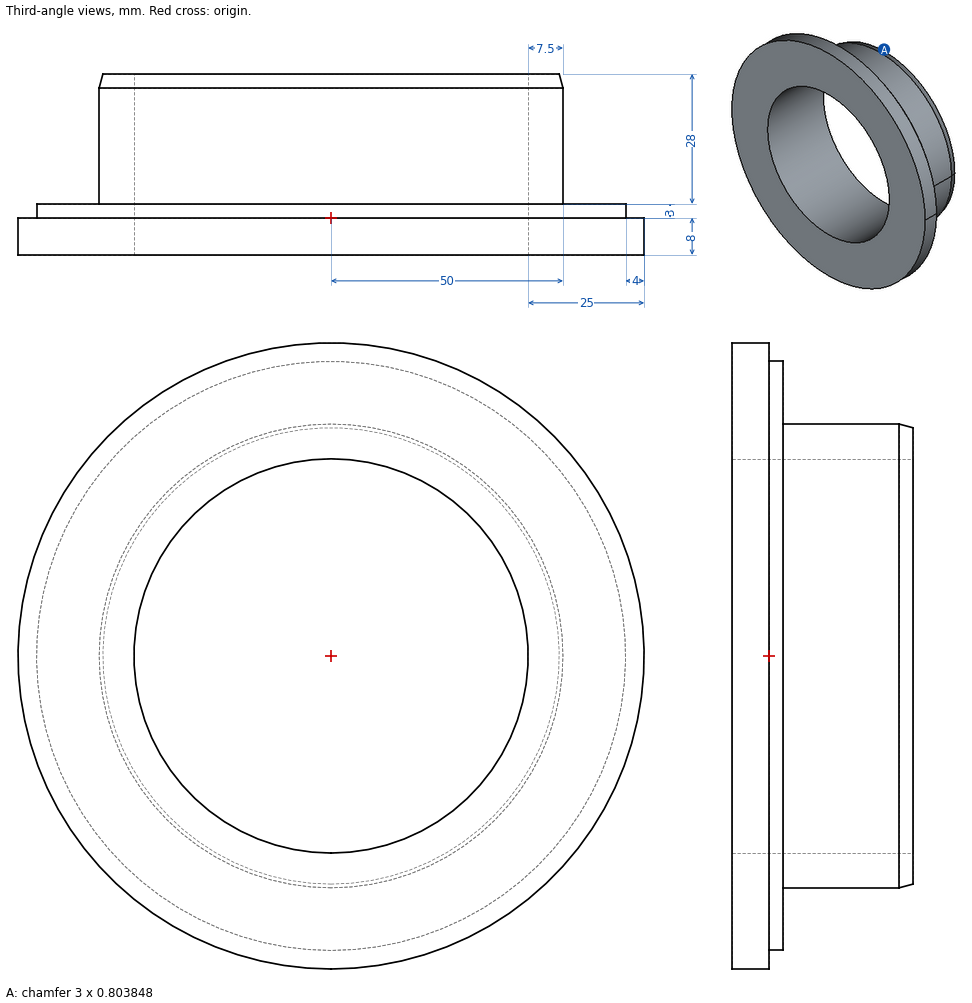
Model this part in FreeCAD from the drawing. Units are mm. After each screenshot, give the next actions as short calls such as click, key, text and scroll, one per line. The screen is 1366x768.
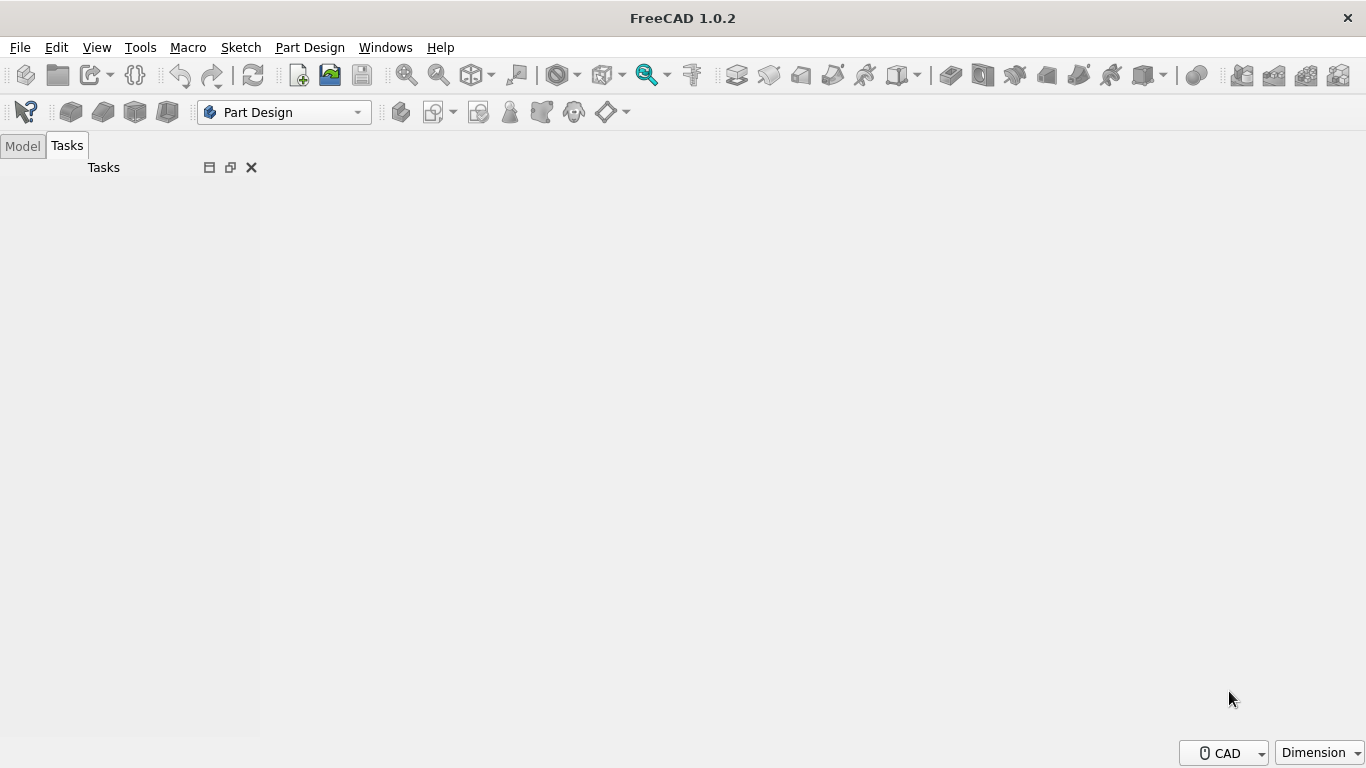
click(298, 76)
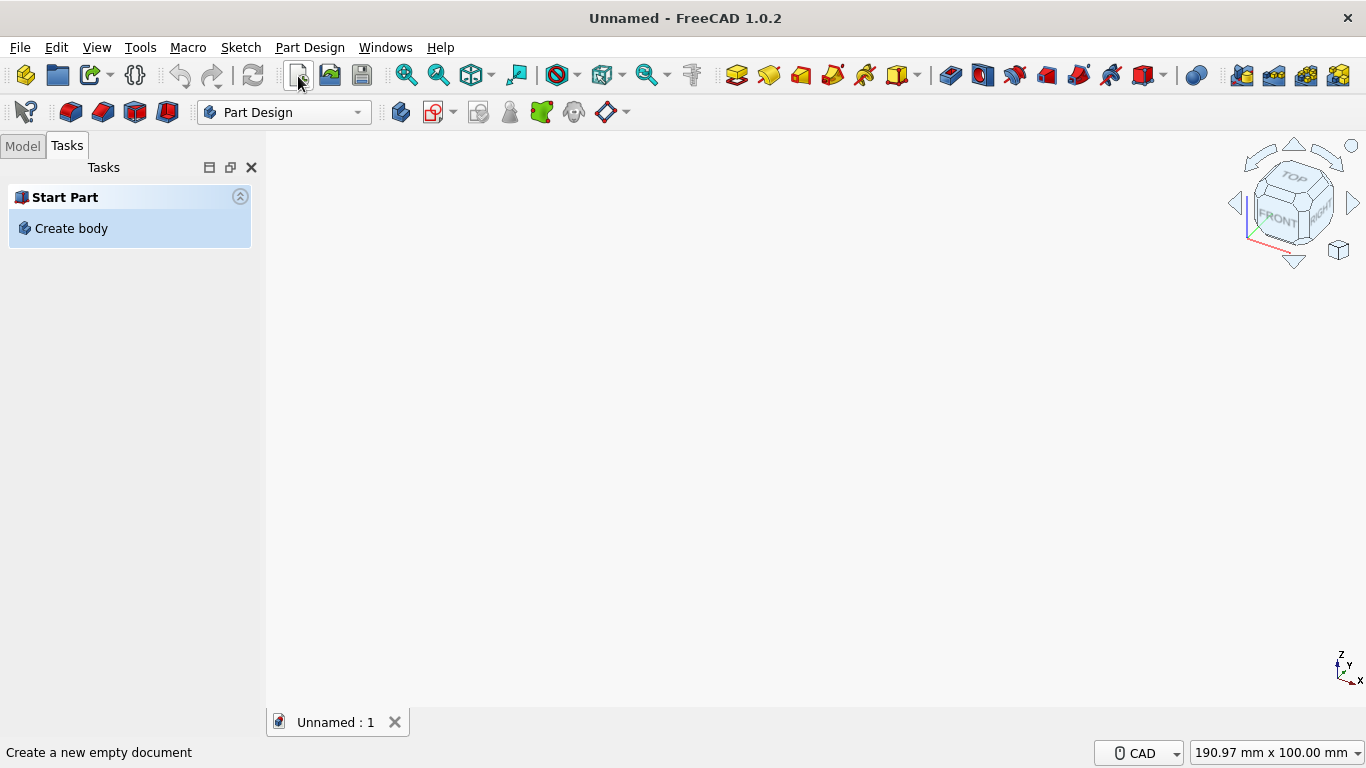
click(434, 112)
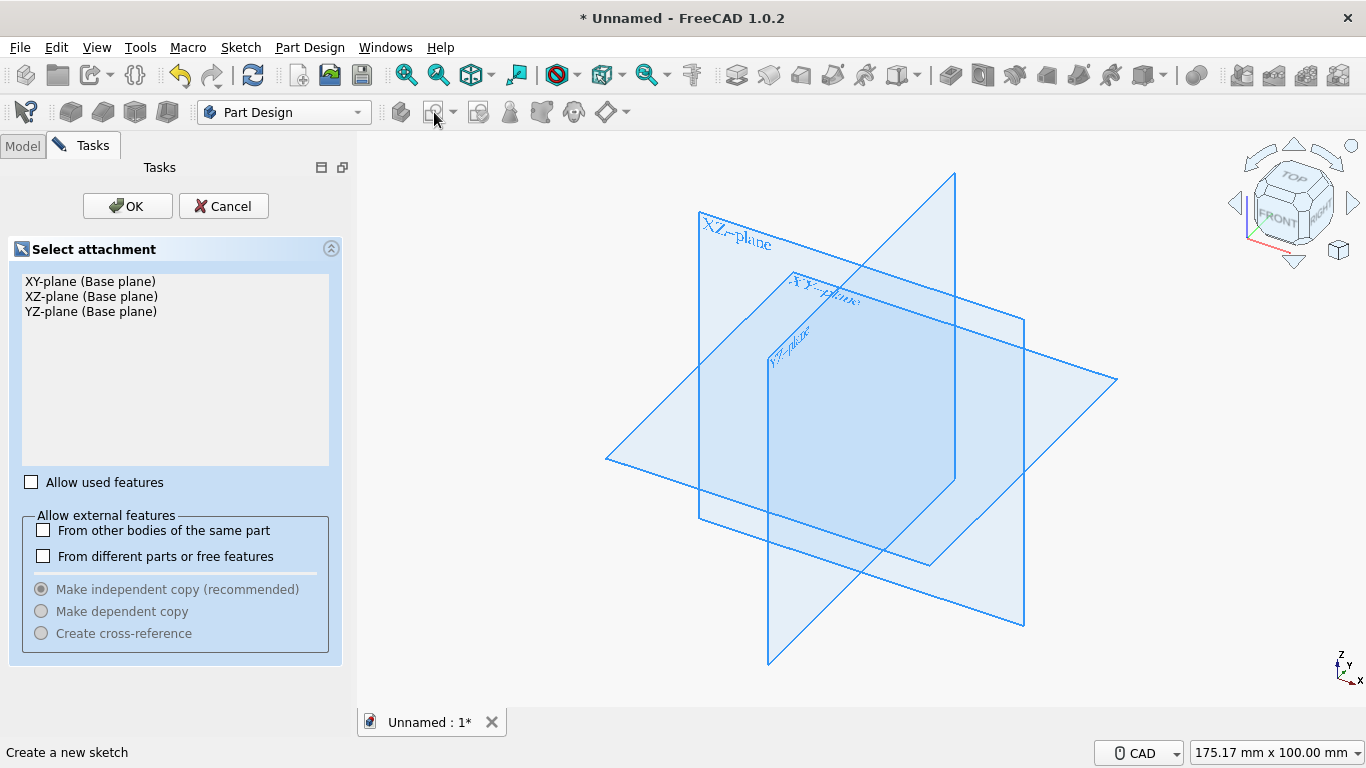
click(82, 282)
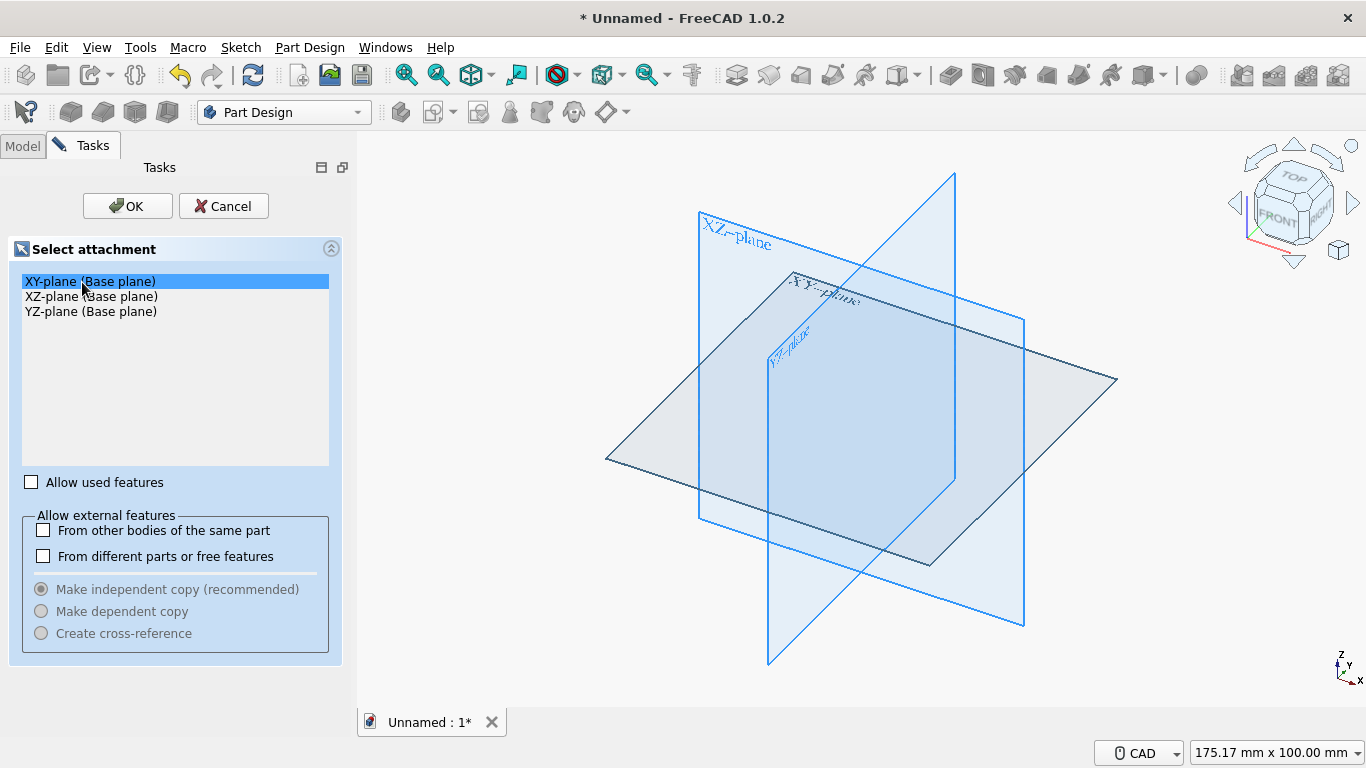
click(128, 206)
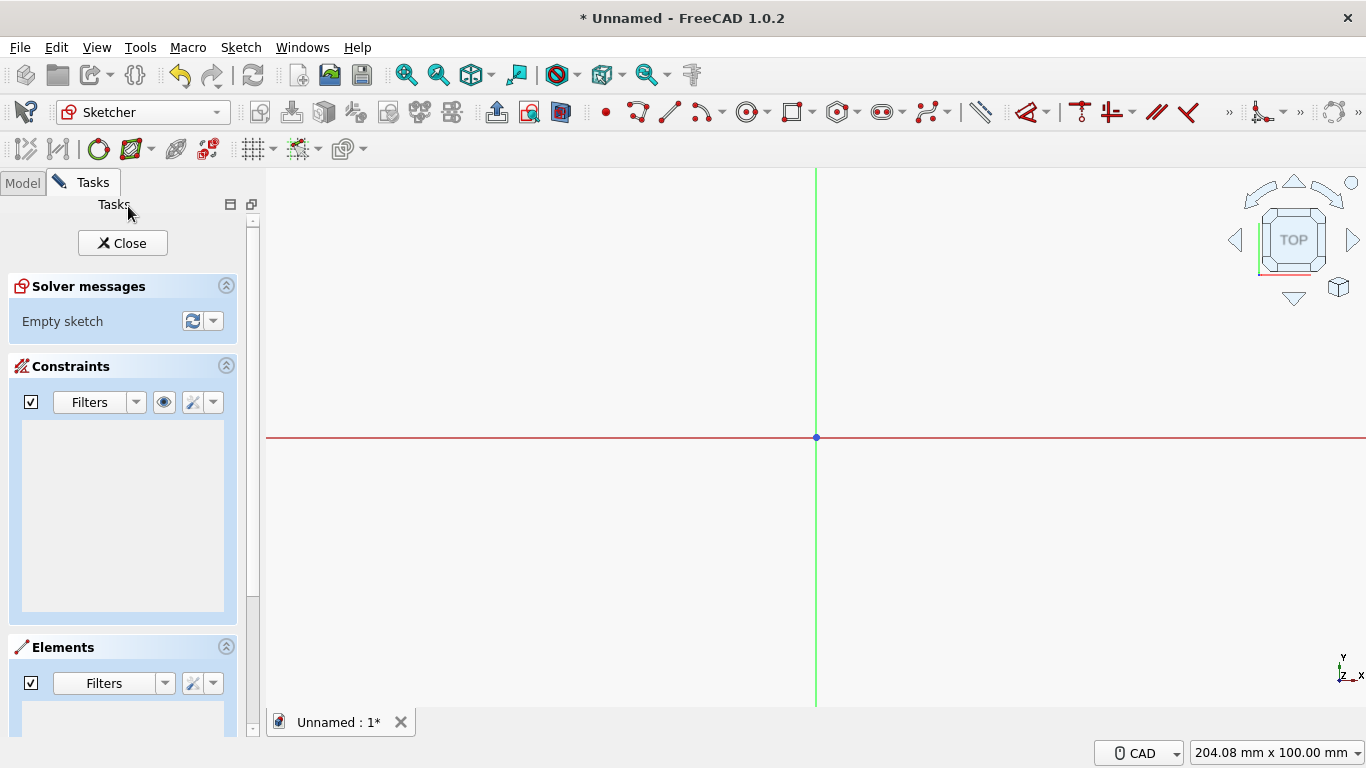
scroll(1201, 249, up, 2)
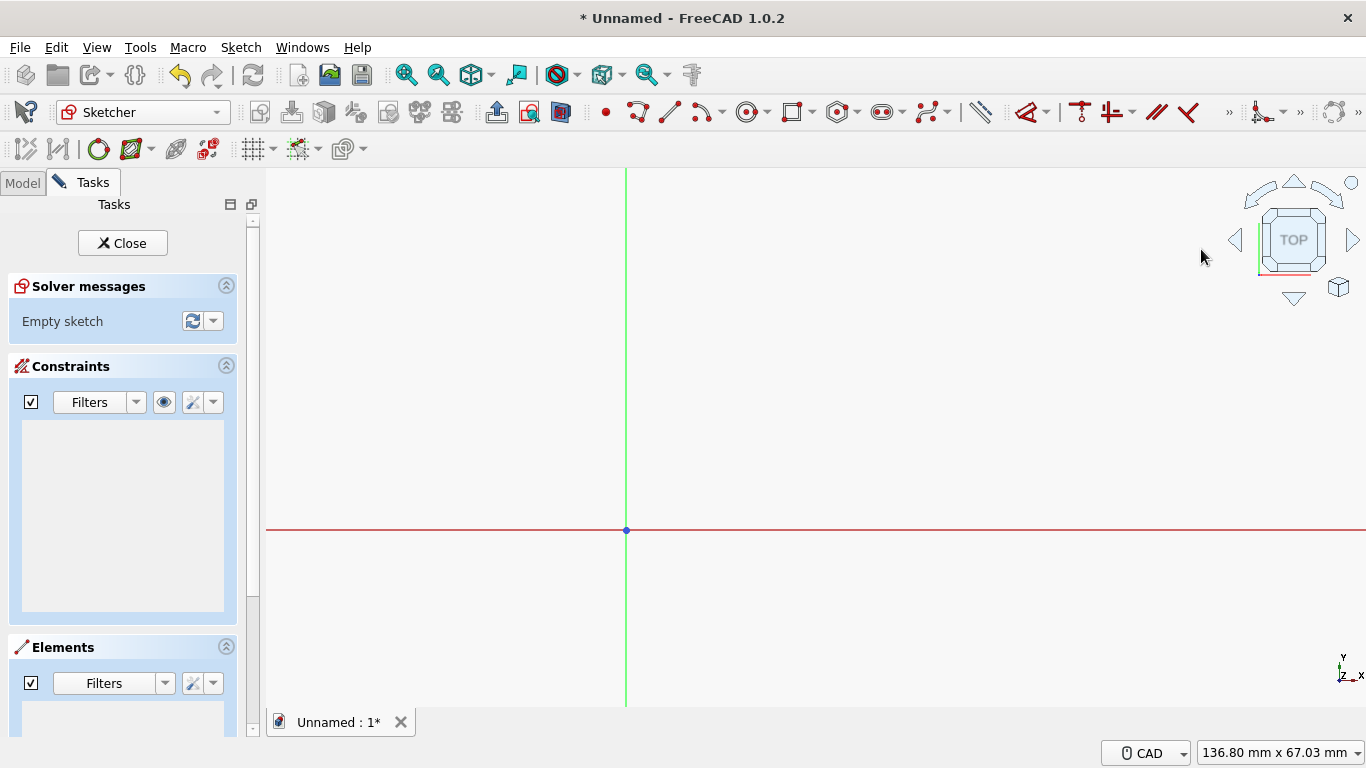
click(638, 112)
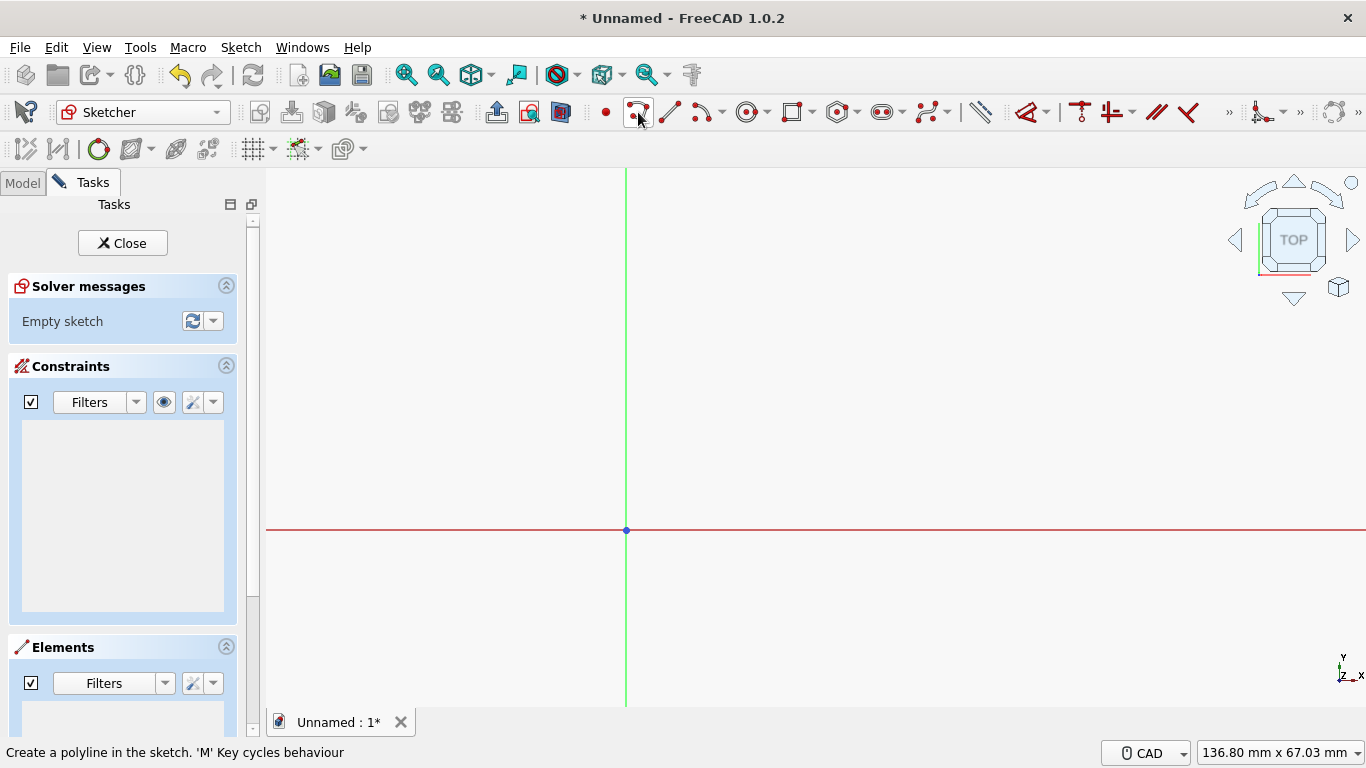
click(968, 594)
click(1169, 594)
click(1169, 530)
click(1137, 521)
click(1137, 506)
click(1028, 506)
click(1028, 281)
click(968, 281)
click(968, 595)
key(Escape)
key(Escape)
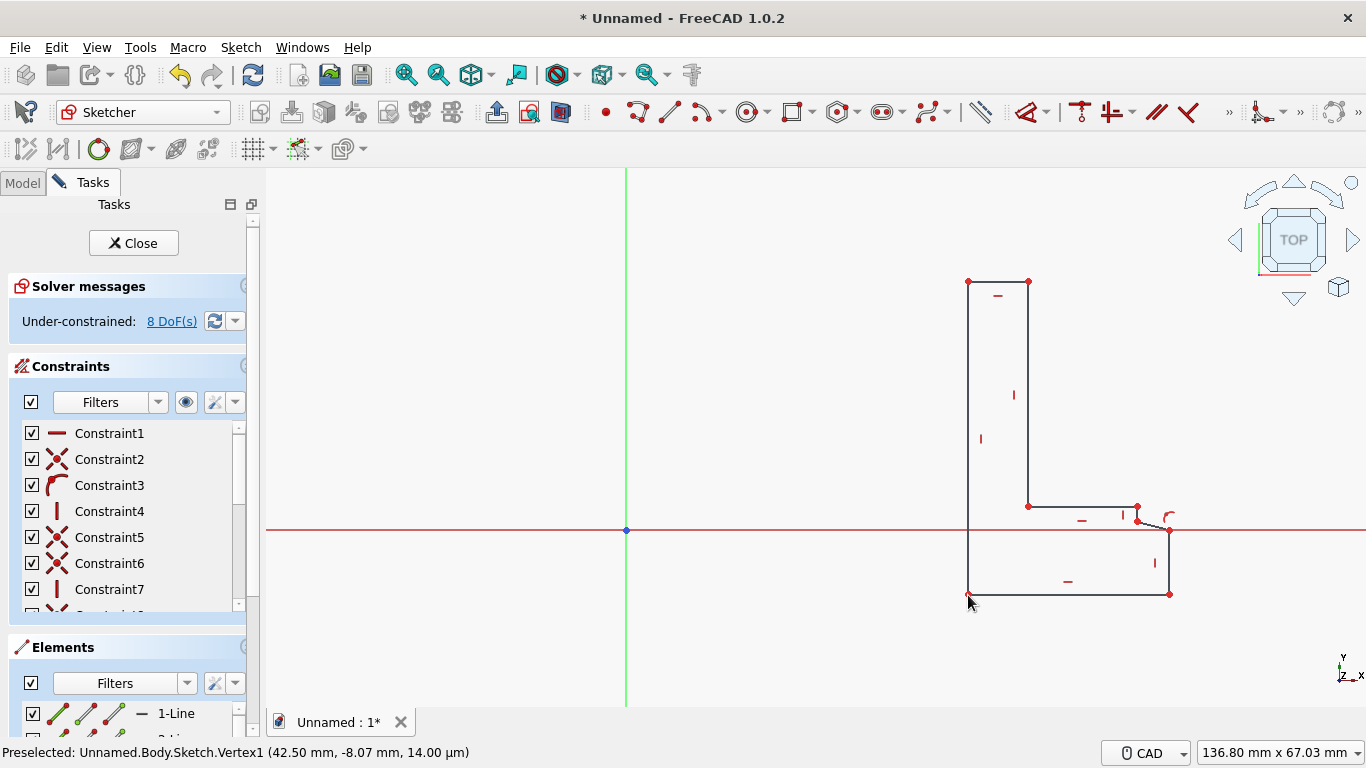
scroll(1159, 528, up, 2)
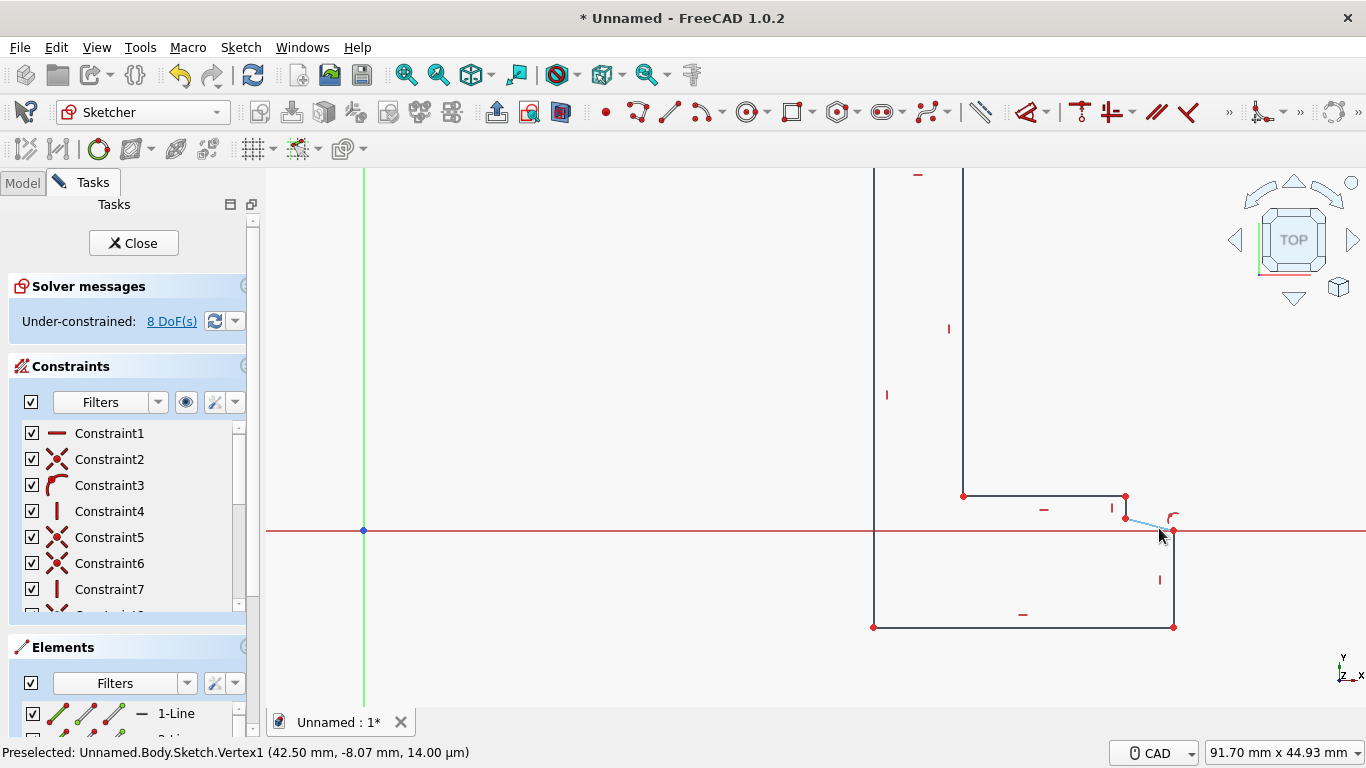
click(1159, 527)